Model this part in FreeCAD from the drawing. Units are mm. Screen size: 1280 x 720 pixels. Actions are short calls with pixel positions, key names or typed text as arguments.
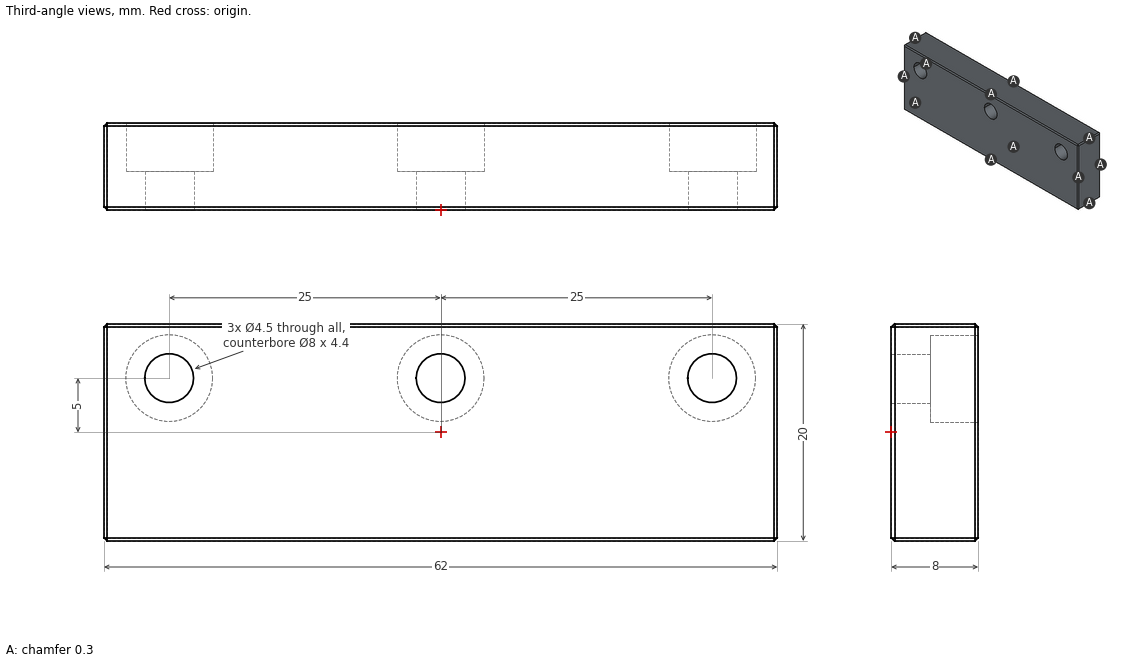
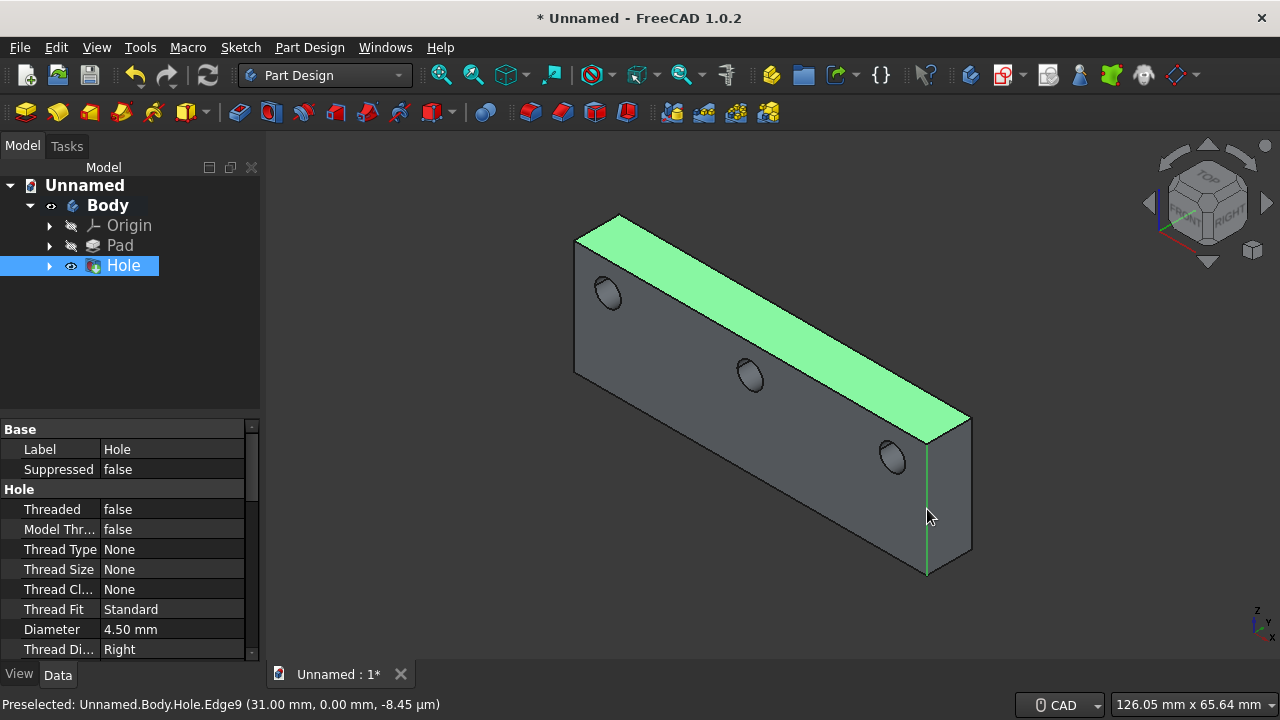
key(2)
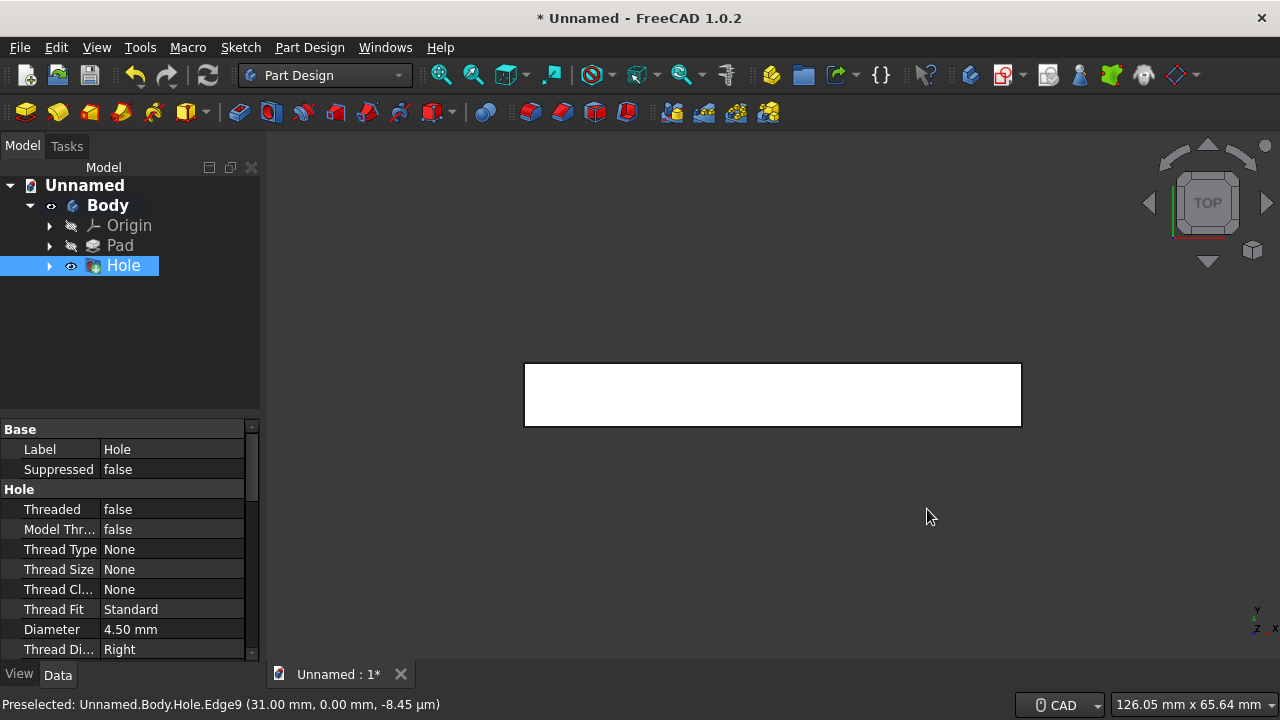
key(1)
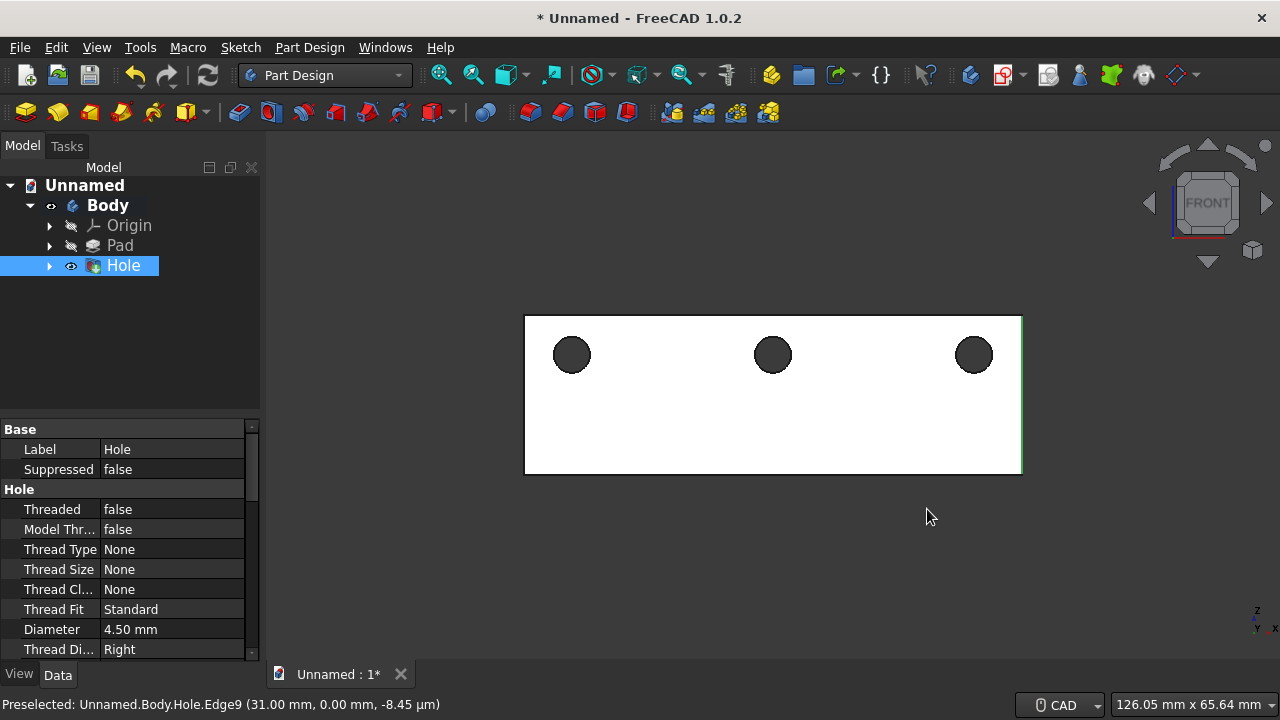
key(3)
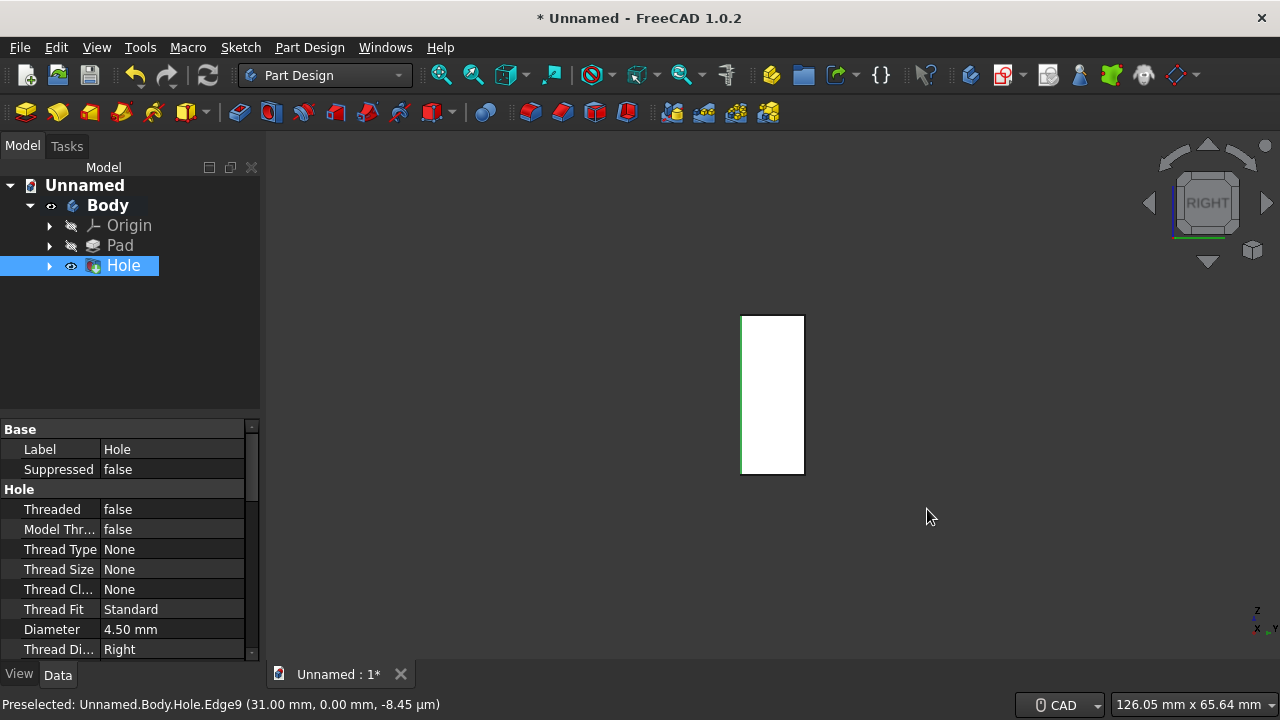
key(v)
key(f)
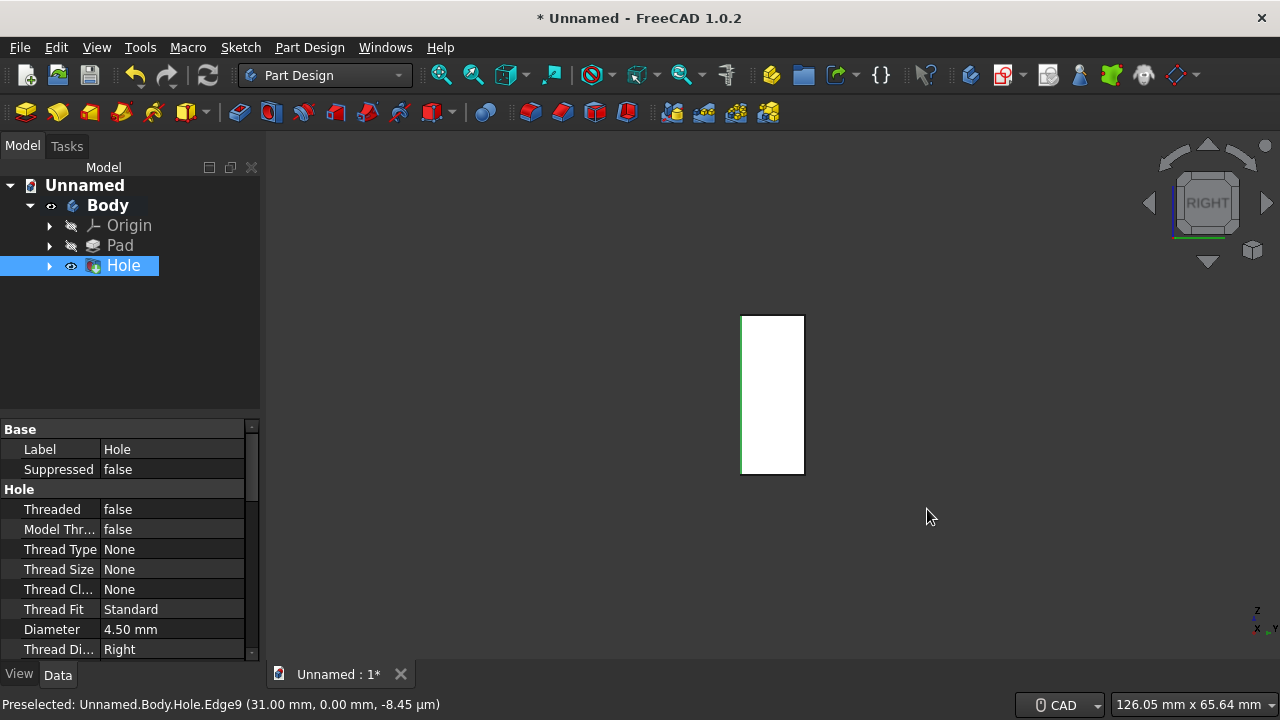
click(805, 394, ctrl)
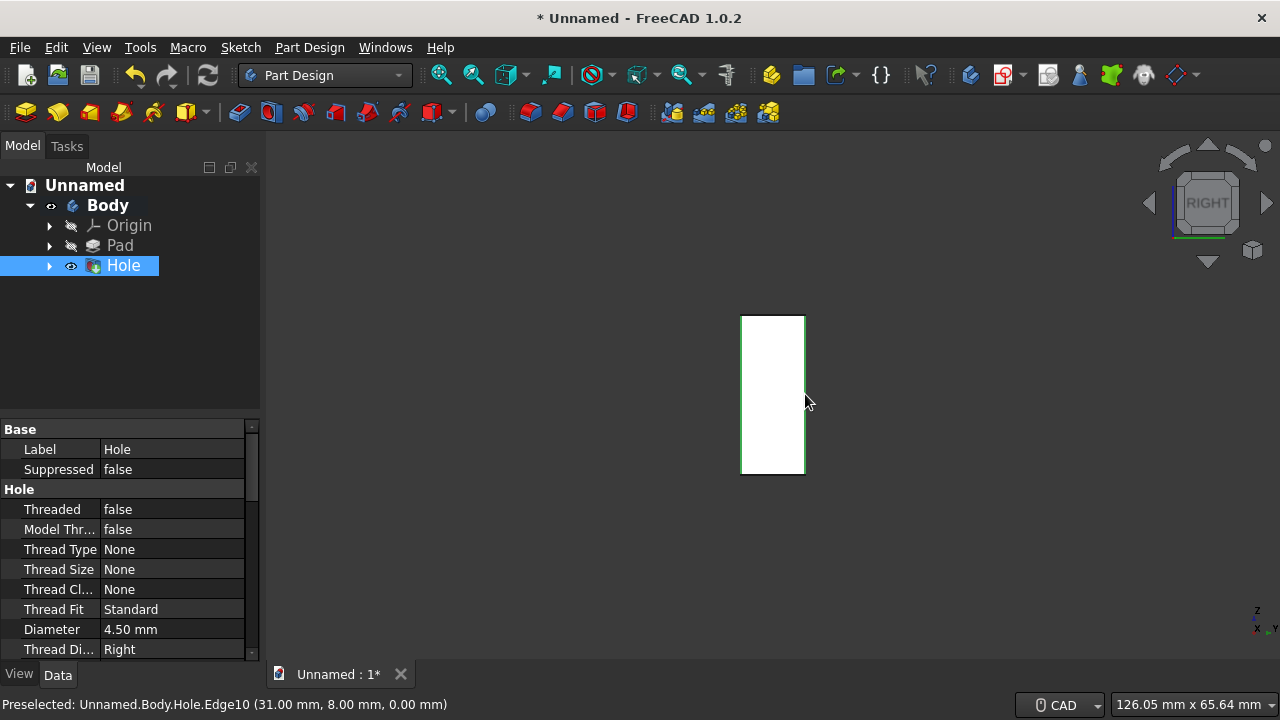
key(5)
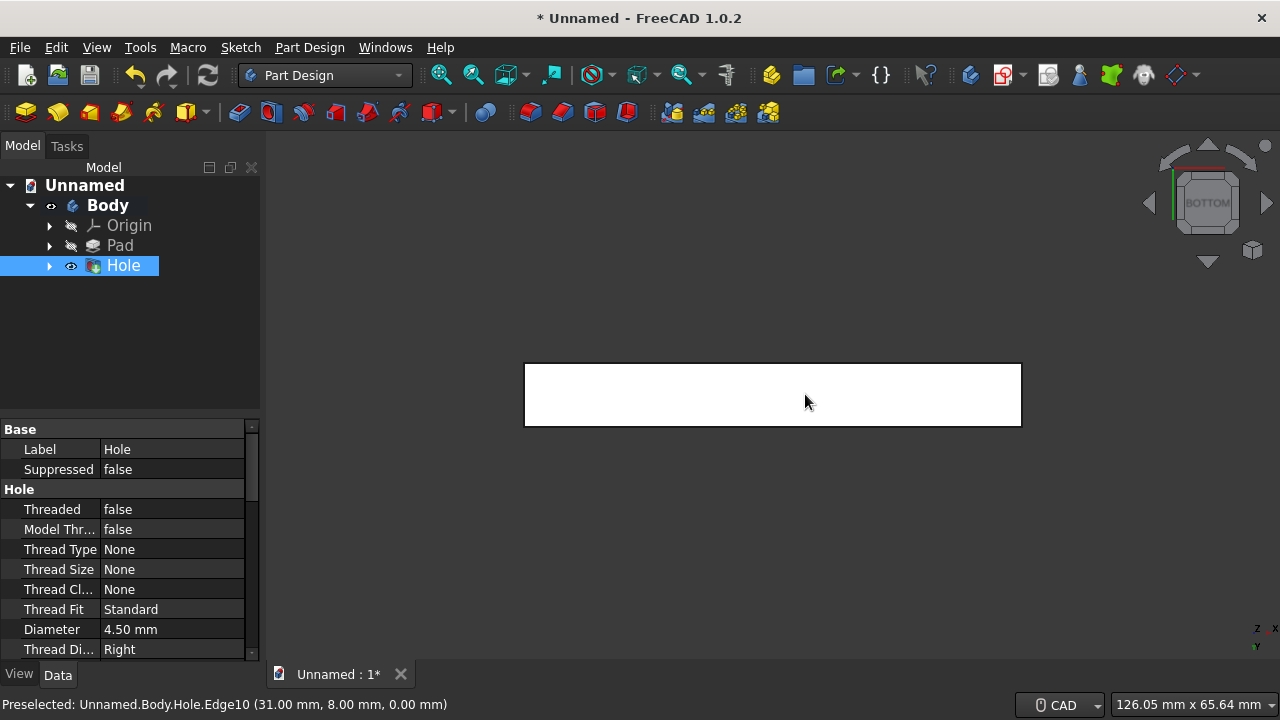
click(987, 394, ctrl)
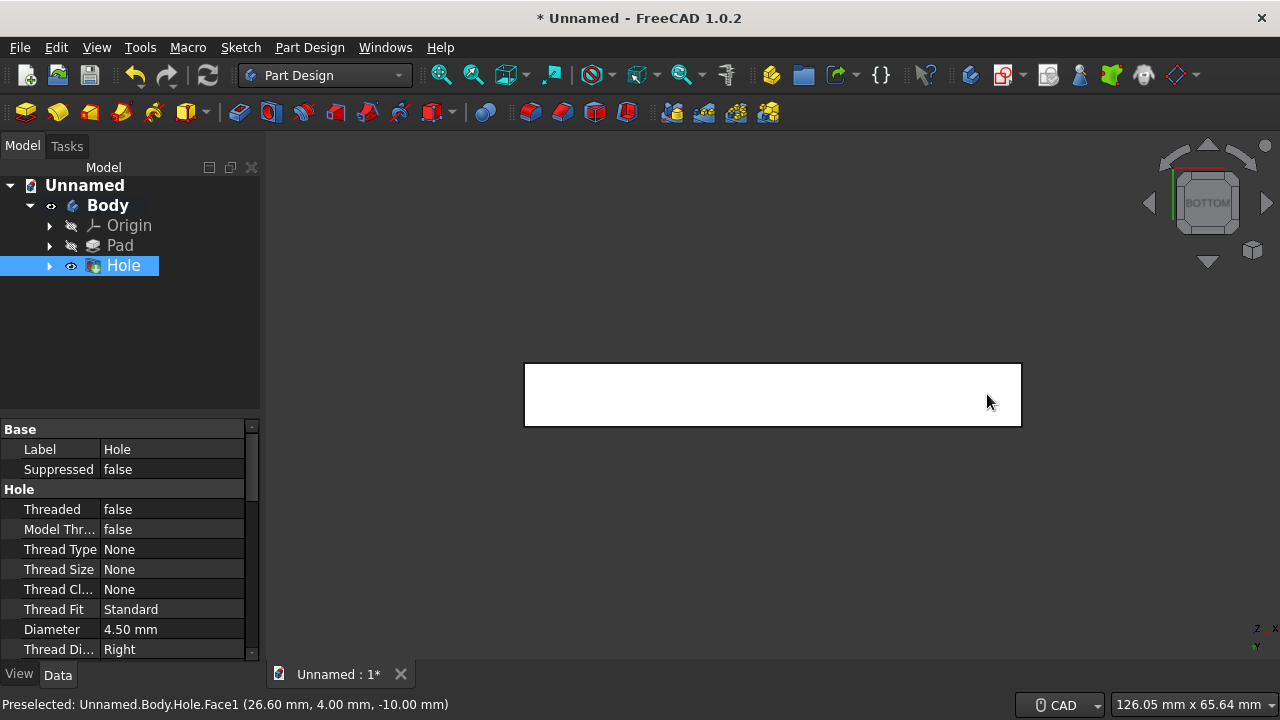
key(4)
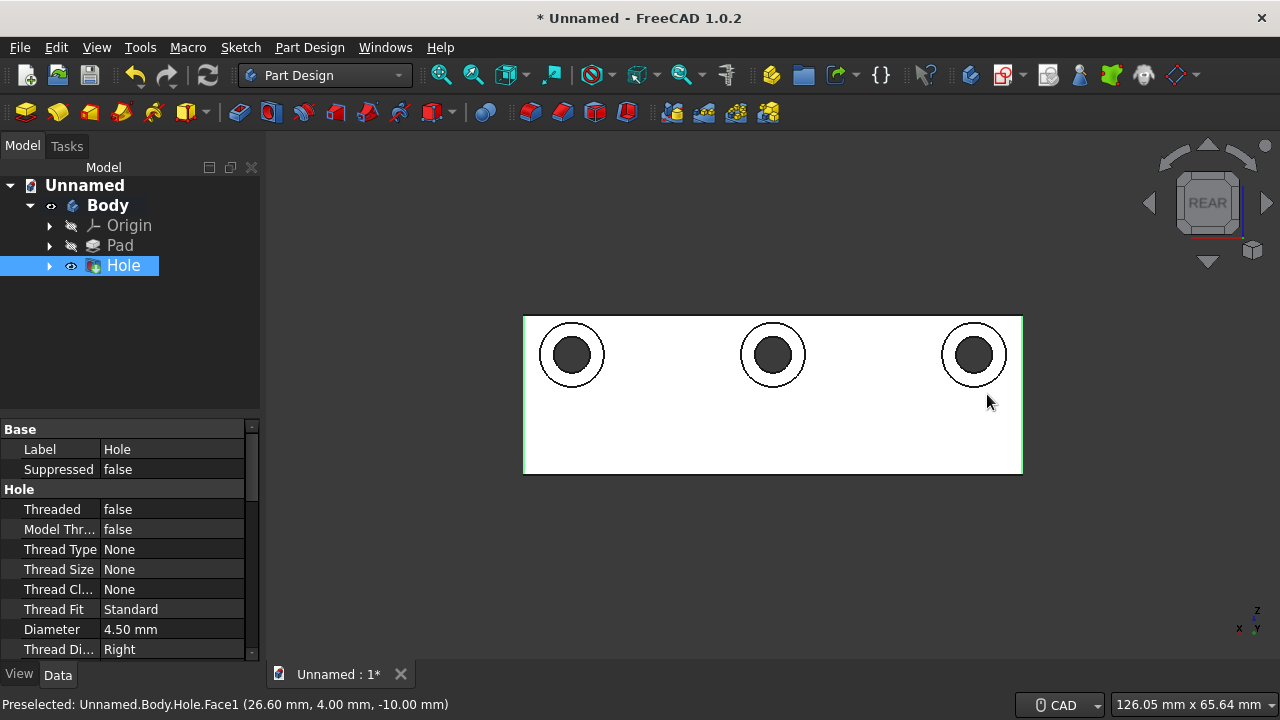
key(6)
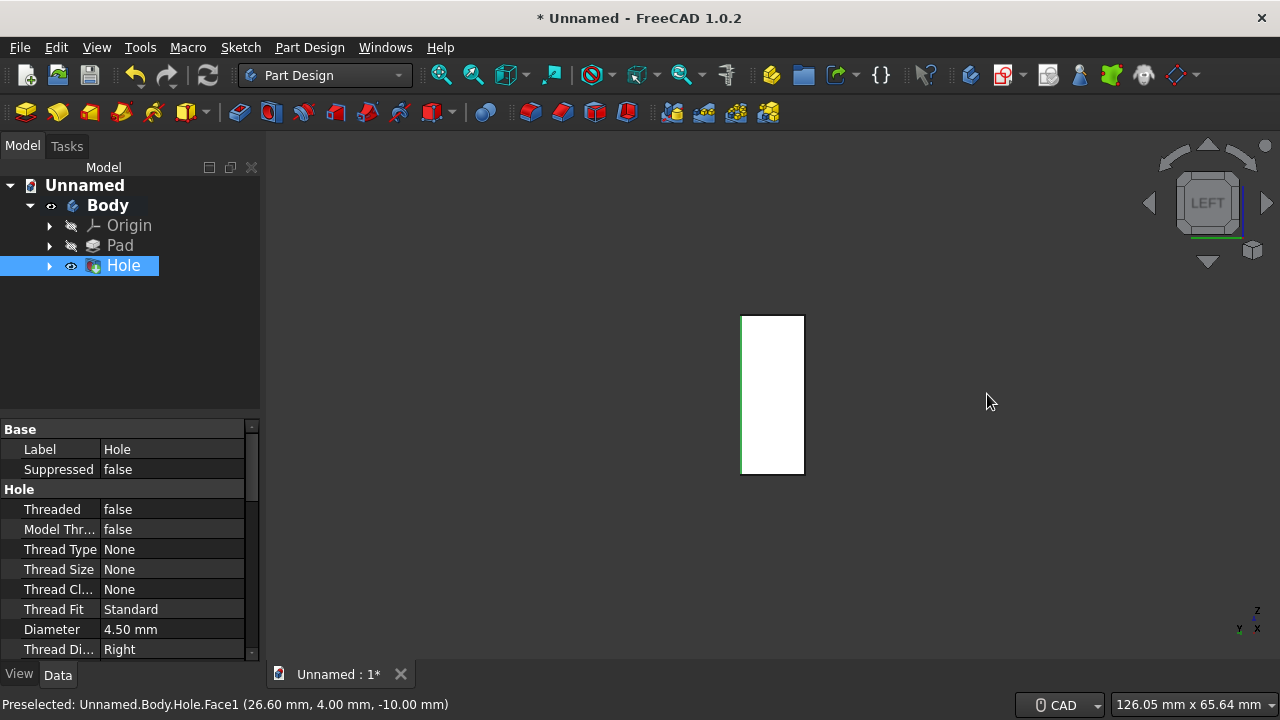
click(442, 76)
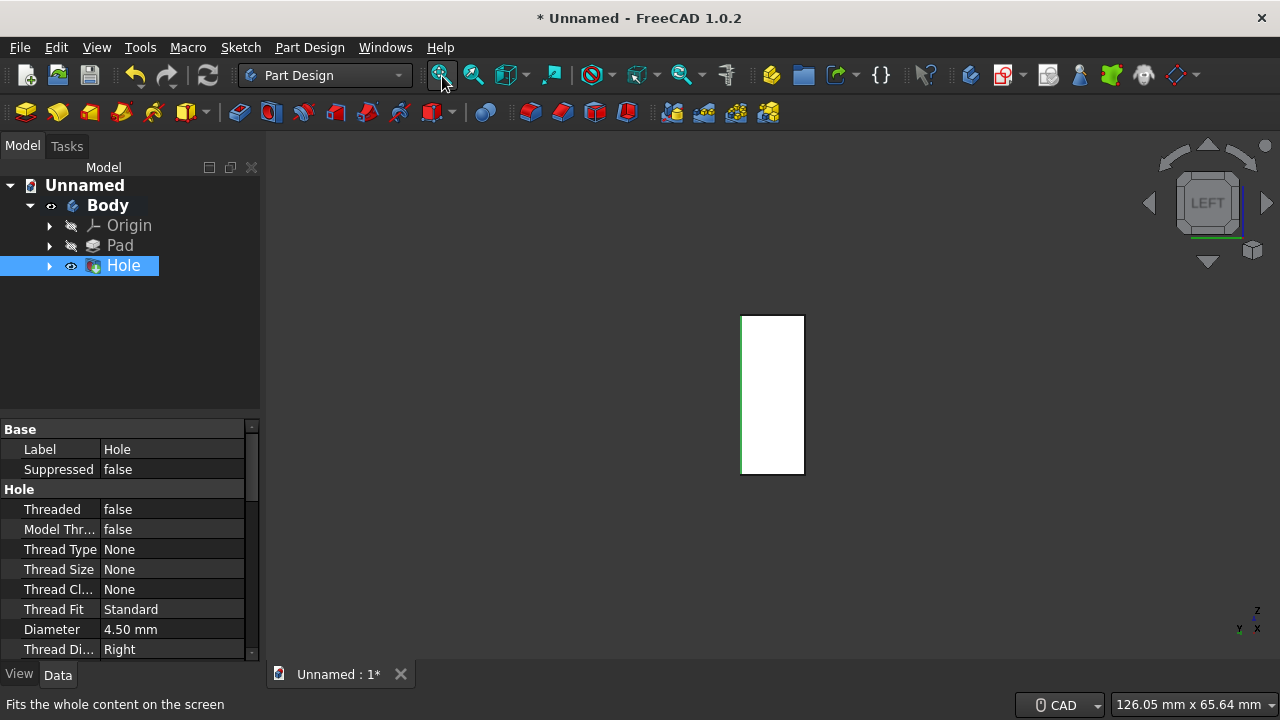
click(805, 394, ctrl)